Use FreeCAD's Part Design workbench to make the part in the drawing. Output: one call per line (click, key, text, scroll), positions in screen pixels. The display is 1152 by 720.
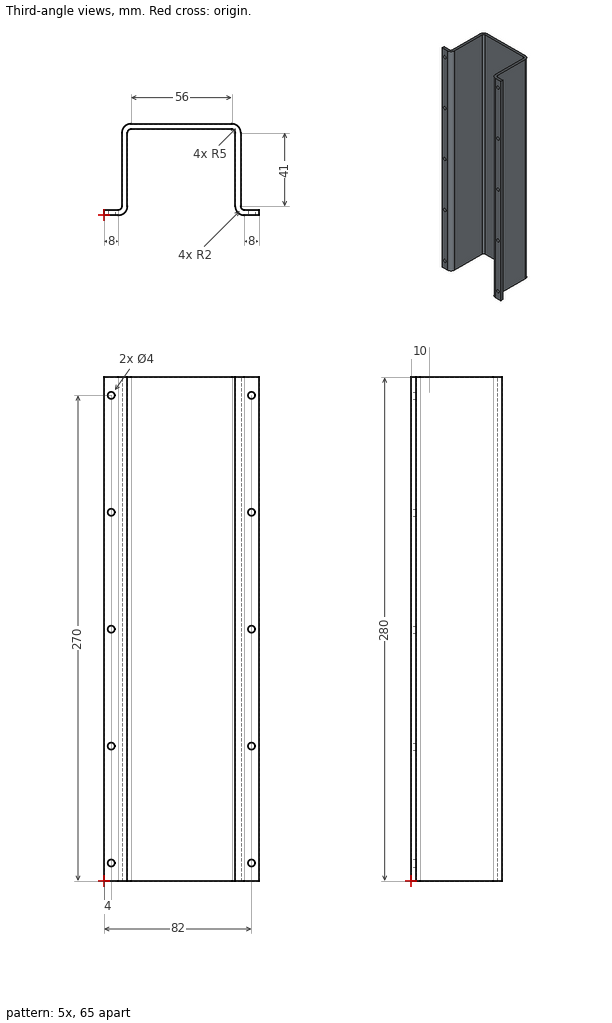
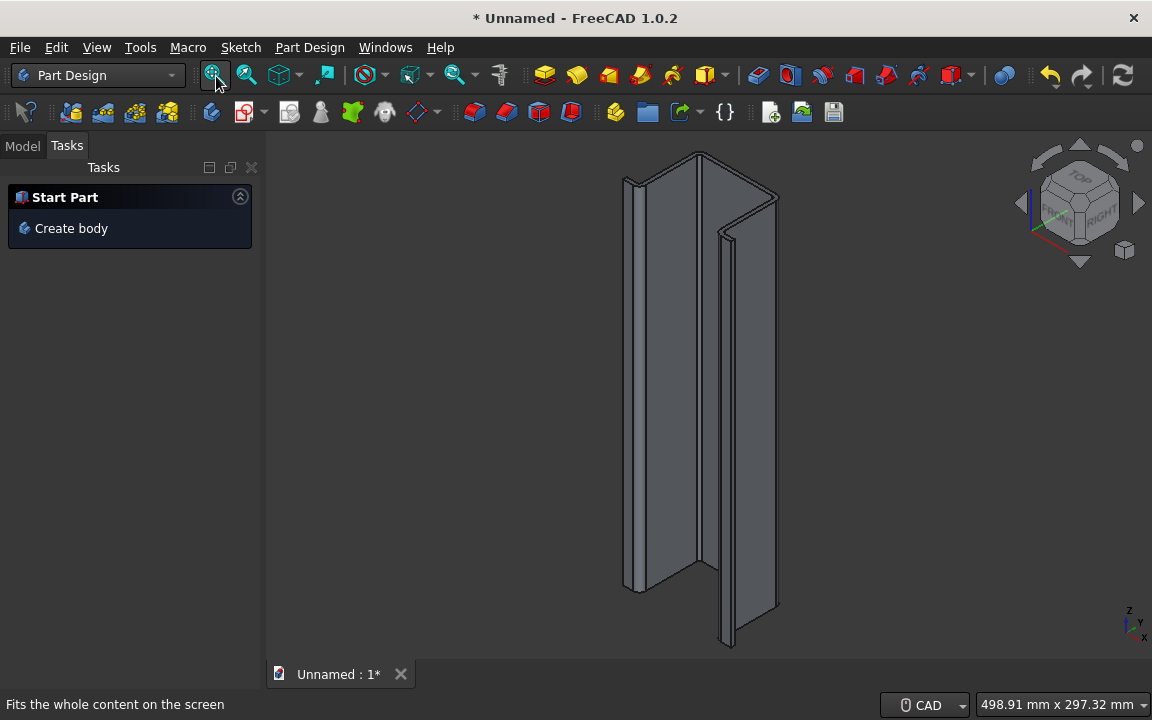
key(1)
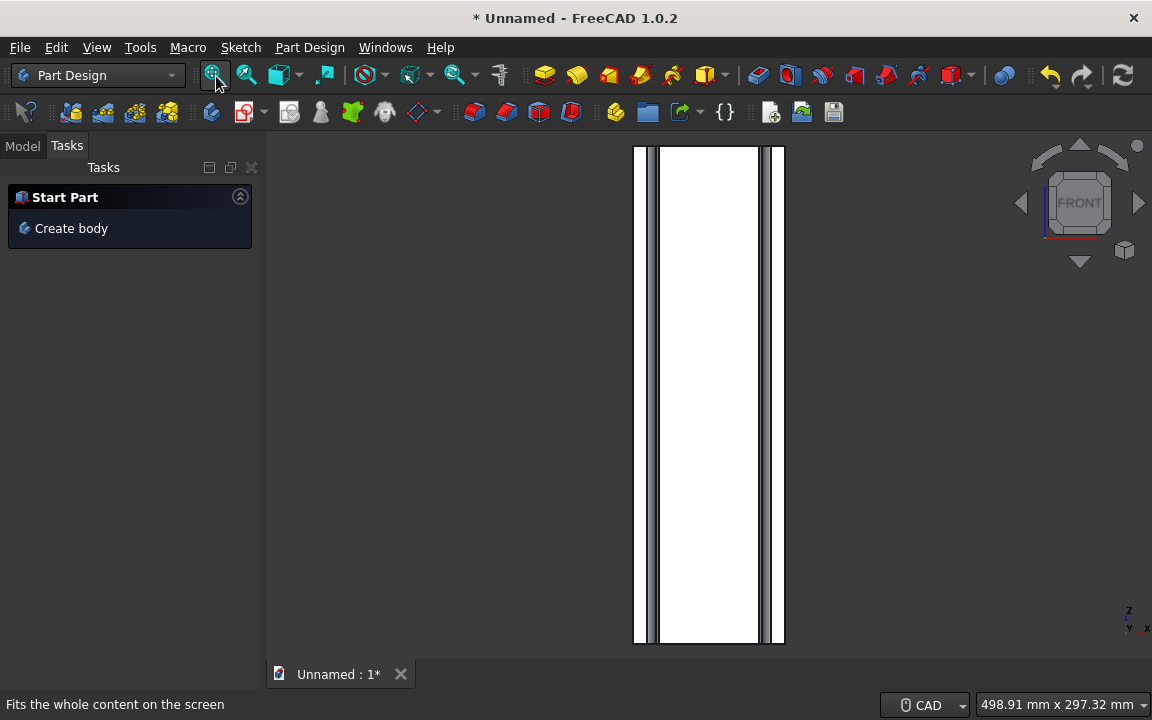
key(2)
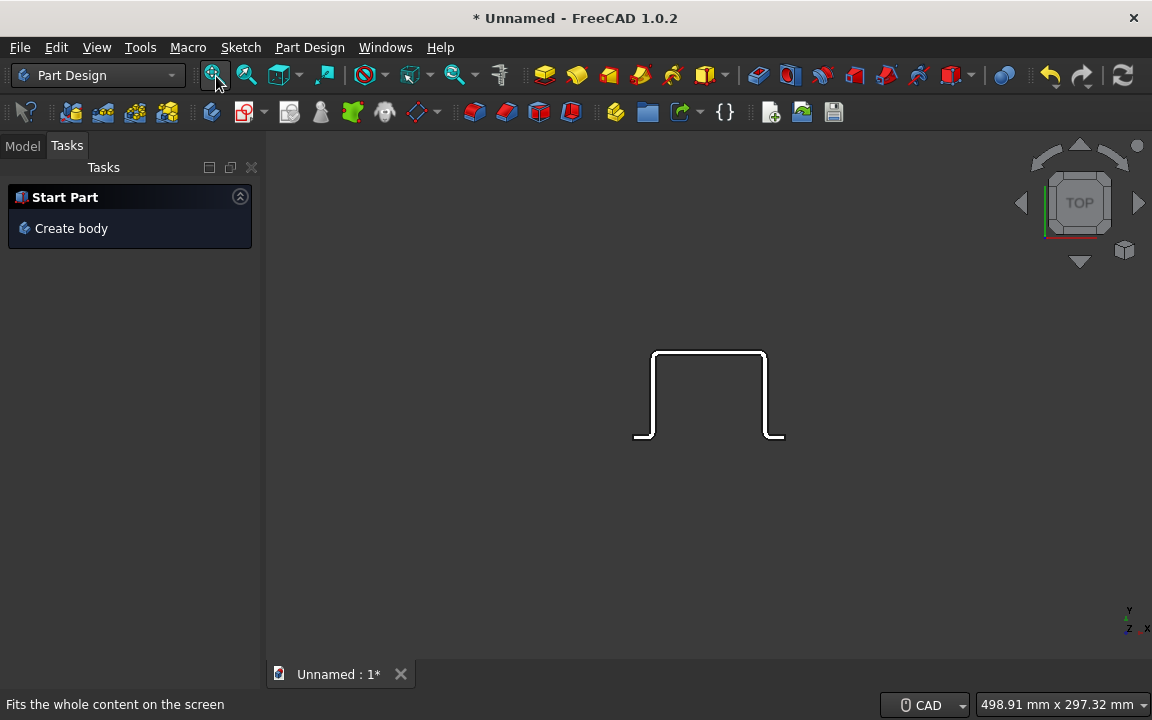
key(v)
key(f)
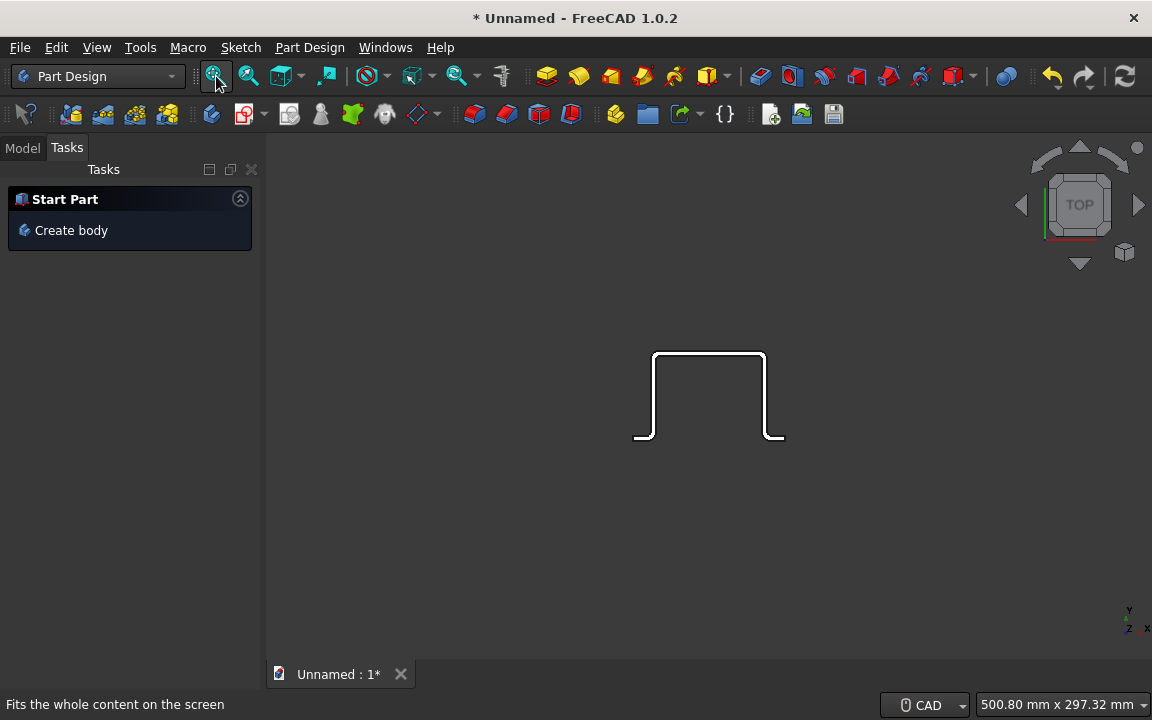
click(244, 114)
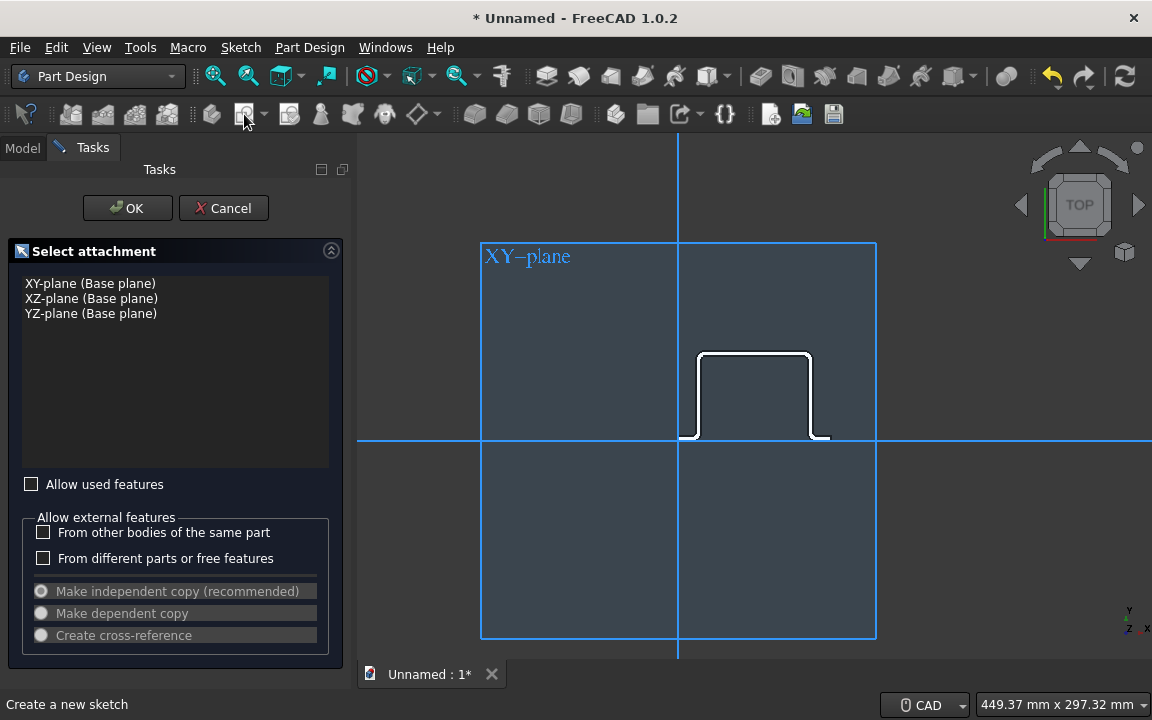
click(82, 298)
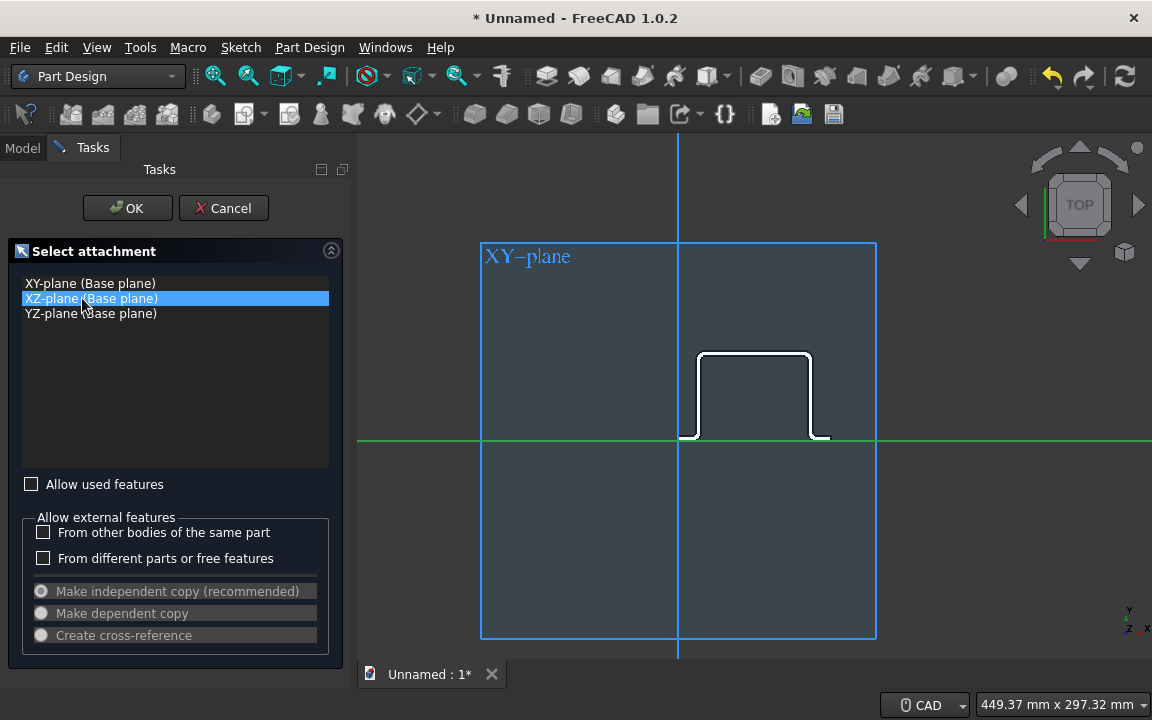
click(128, 208)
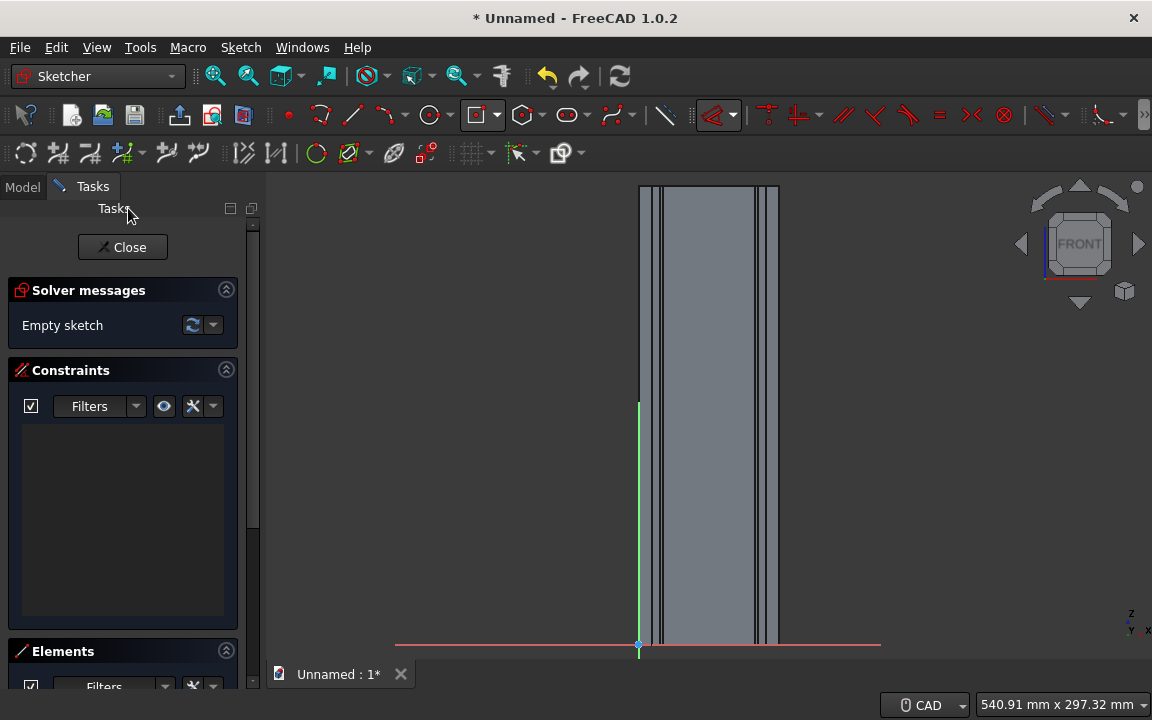
scroll(640, 416, down, 5)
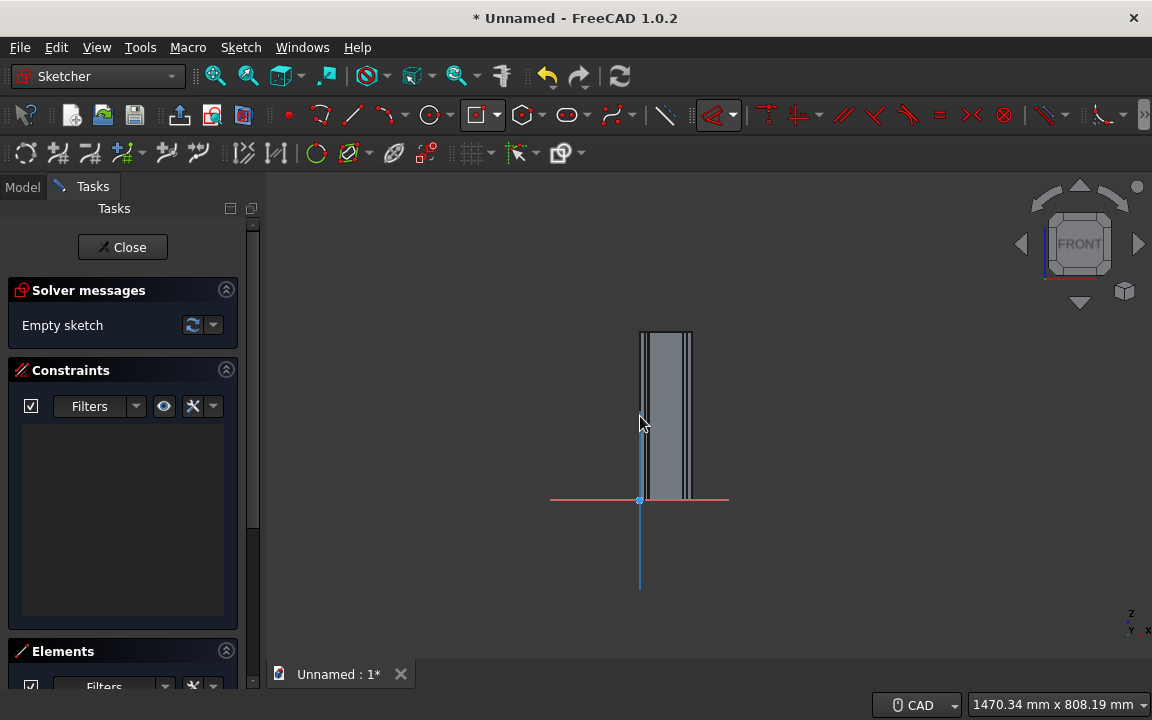
scroll(669, 328, up, 11)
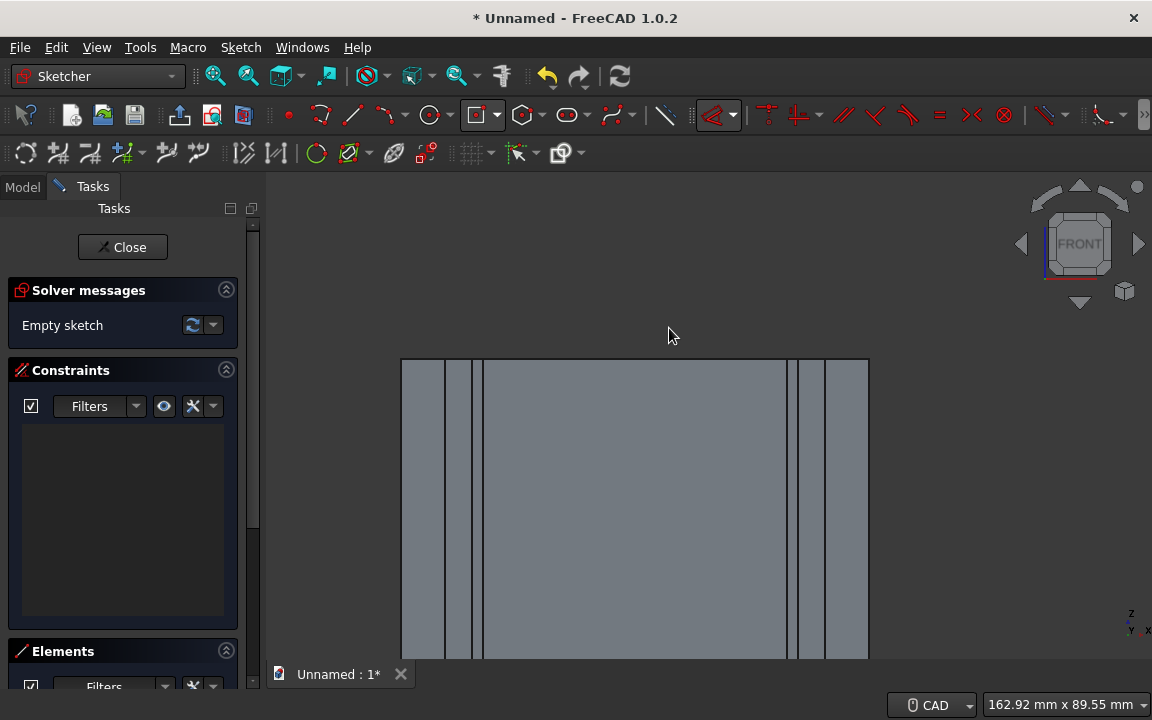
key(g)
key(c)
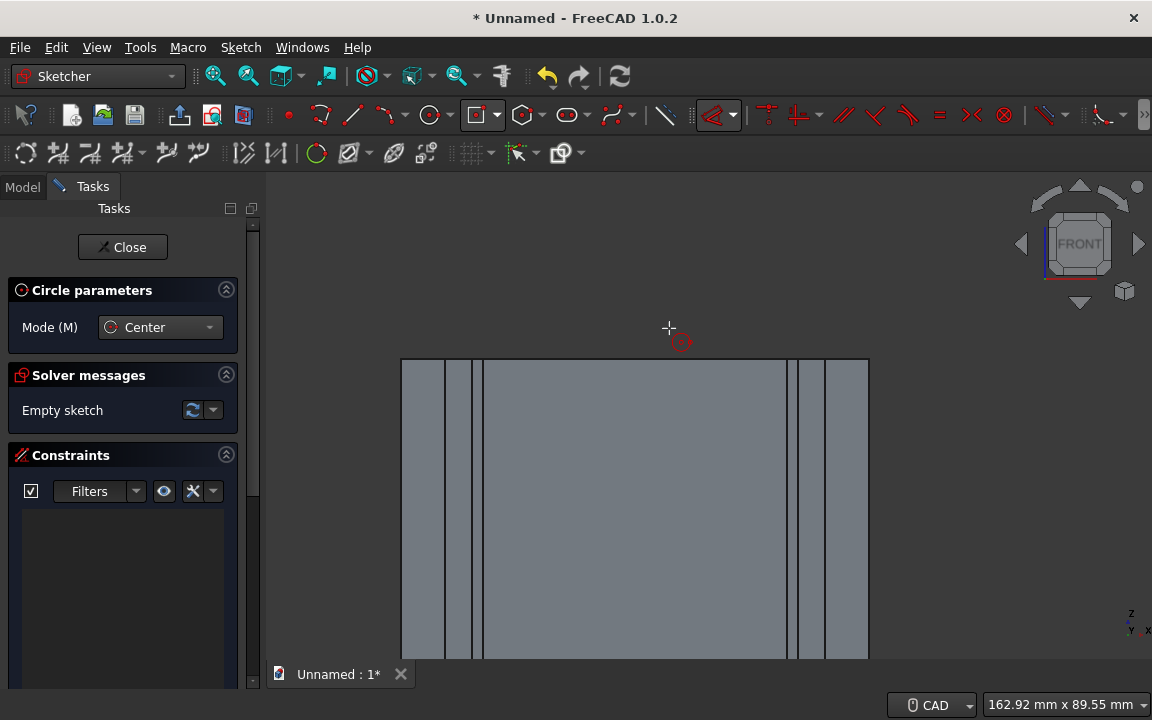
scroll(423, 414, up, 4)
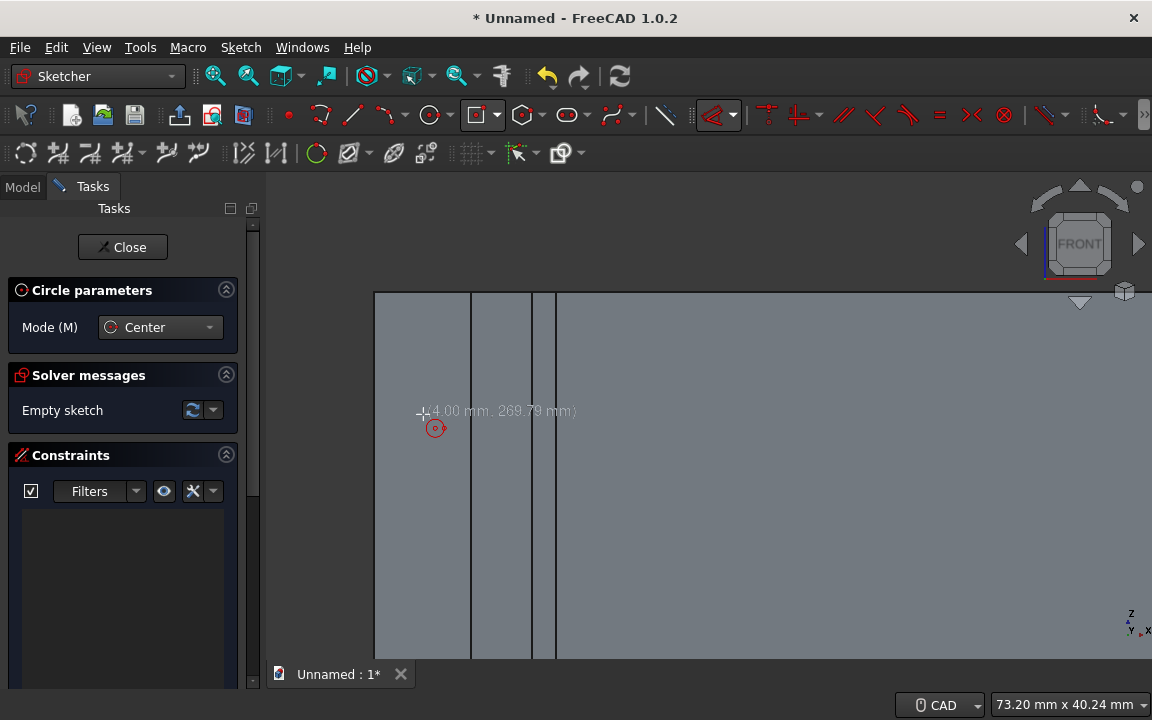
click(423, 413)
click(440, 396)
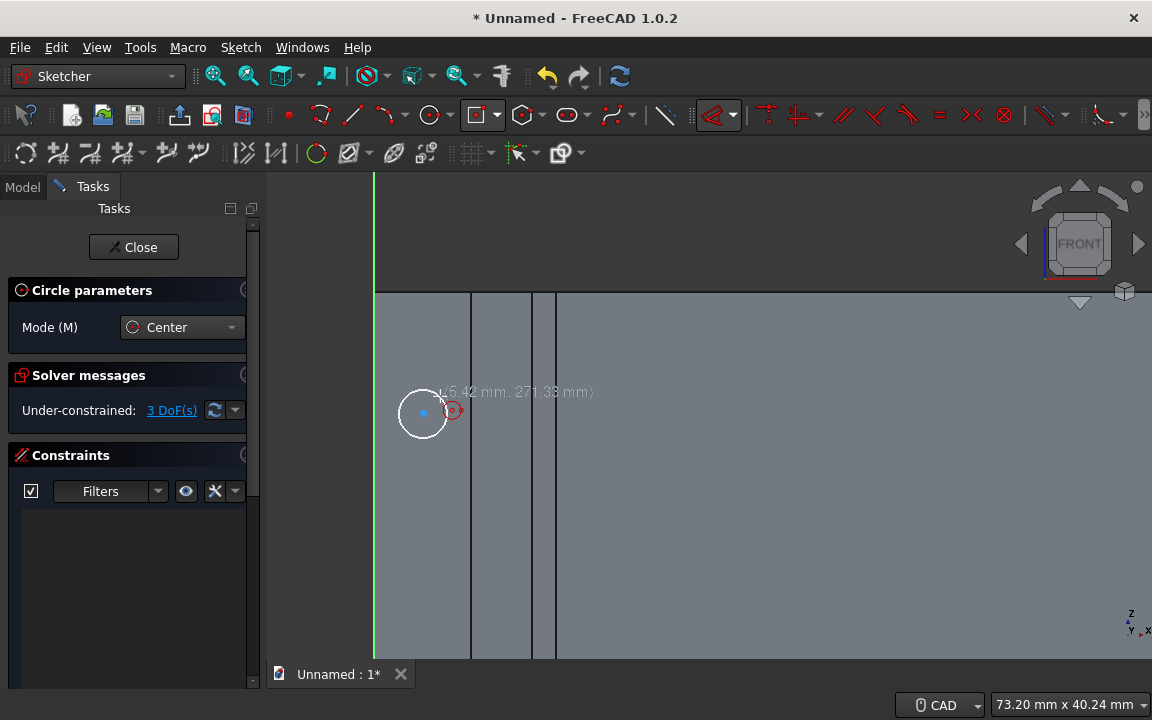
scroll(433, 417, down, 4)